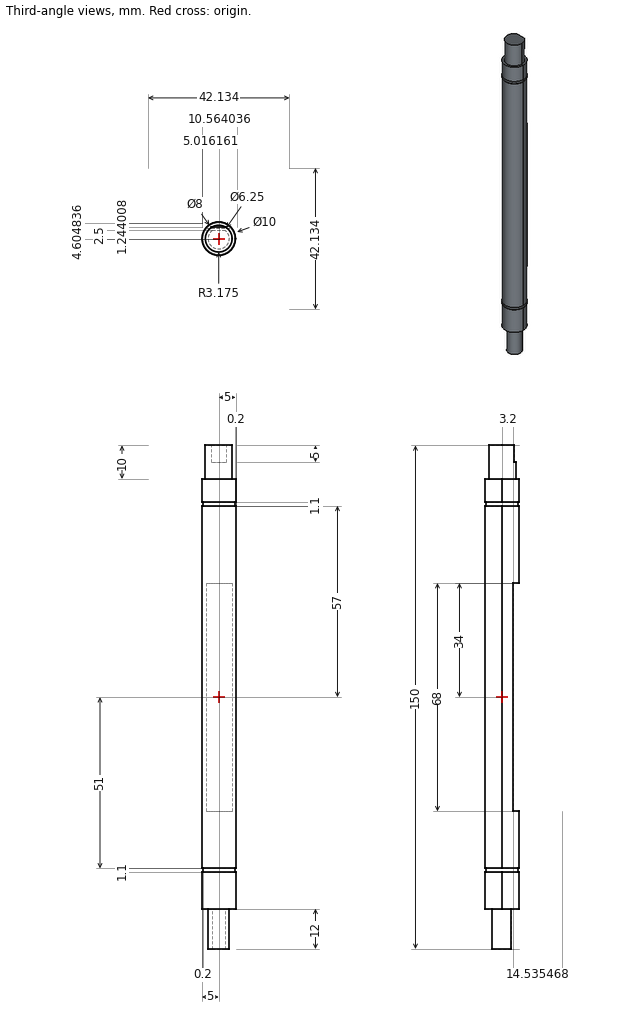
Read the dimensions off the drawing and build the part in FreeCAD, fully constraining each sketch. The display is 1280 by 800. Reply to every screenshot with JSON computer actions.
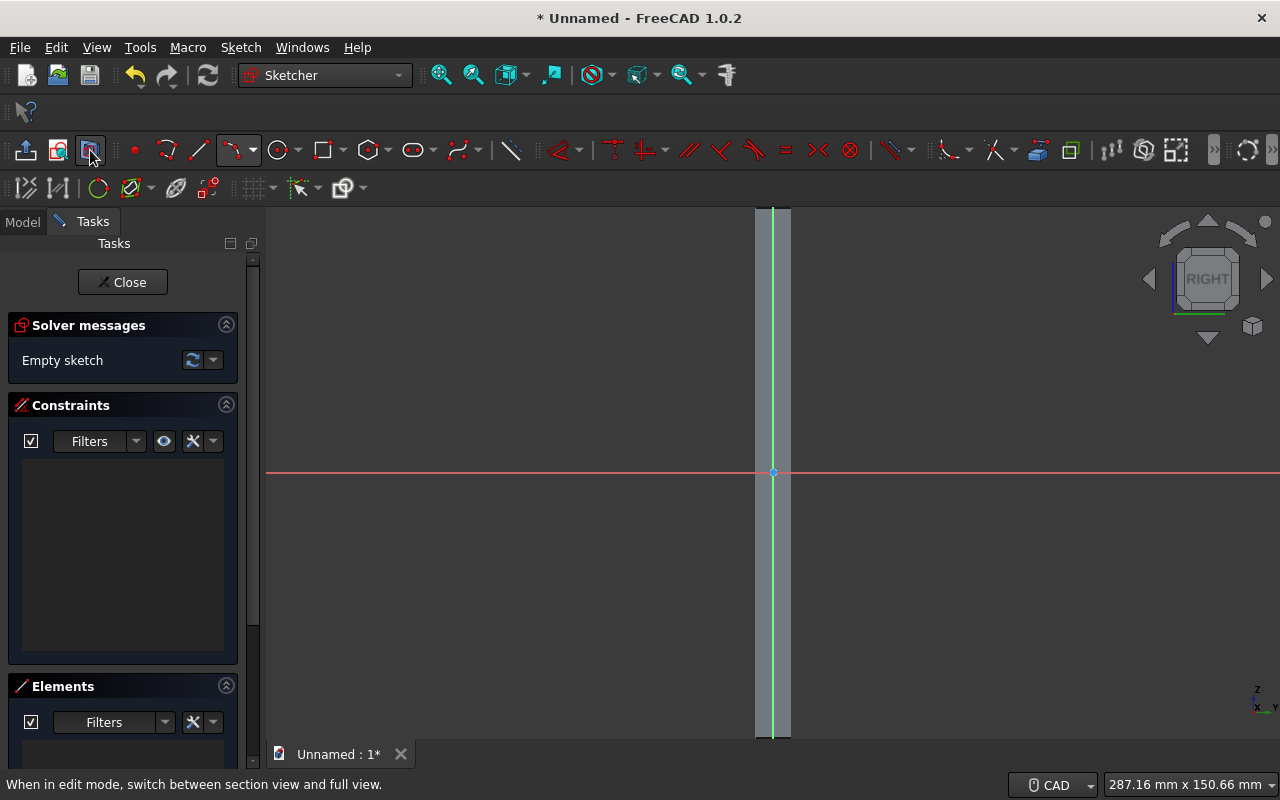
{"action": "scroll", "coordinate": [1007, 473], "scroll_direction": "up", "scroll_amount": 2}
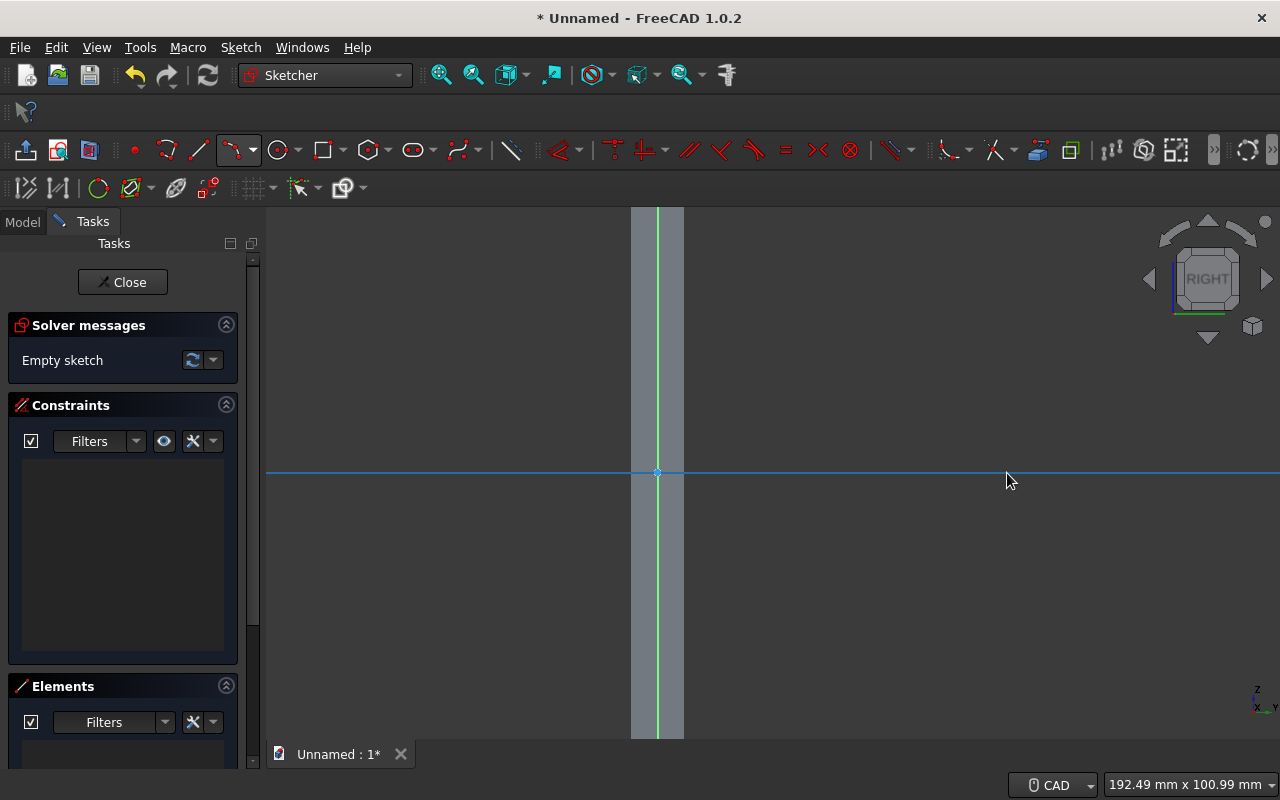
{"action": "key", "text": "g r"}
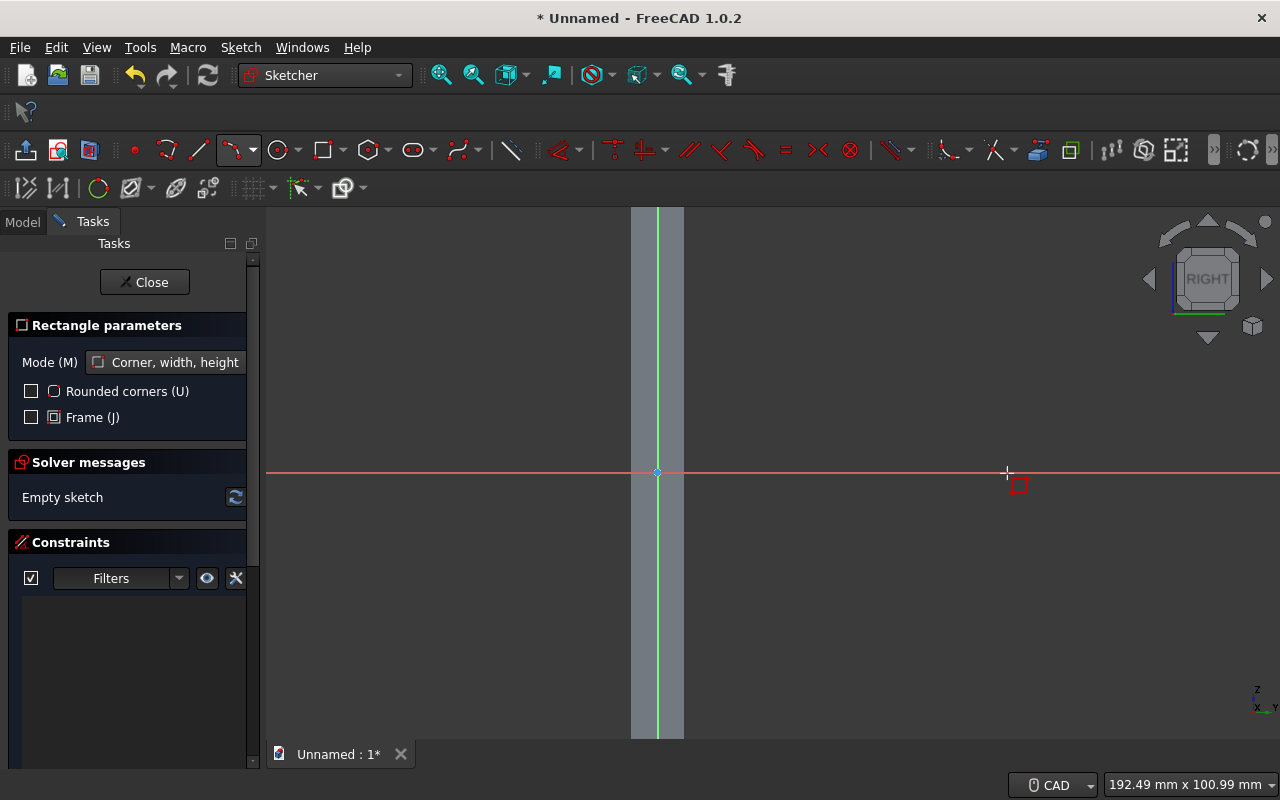
{"action": "left_click", "coordinate": [674, 294]}
{"action": "left_click", "coordinate": [751, 652]}
{"action": "key", "text": "Escape"}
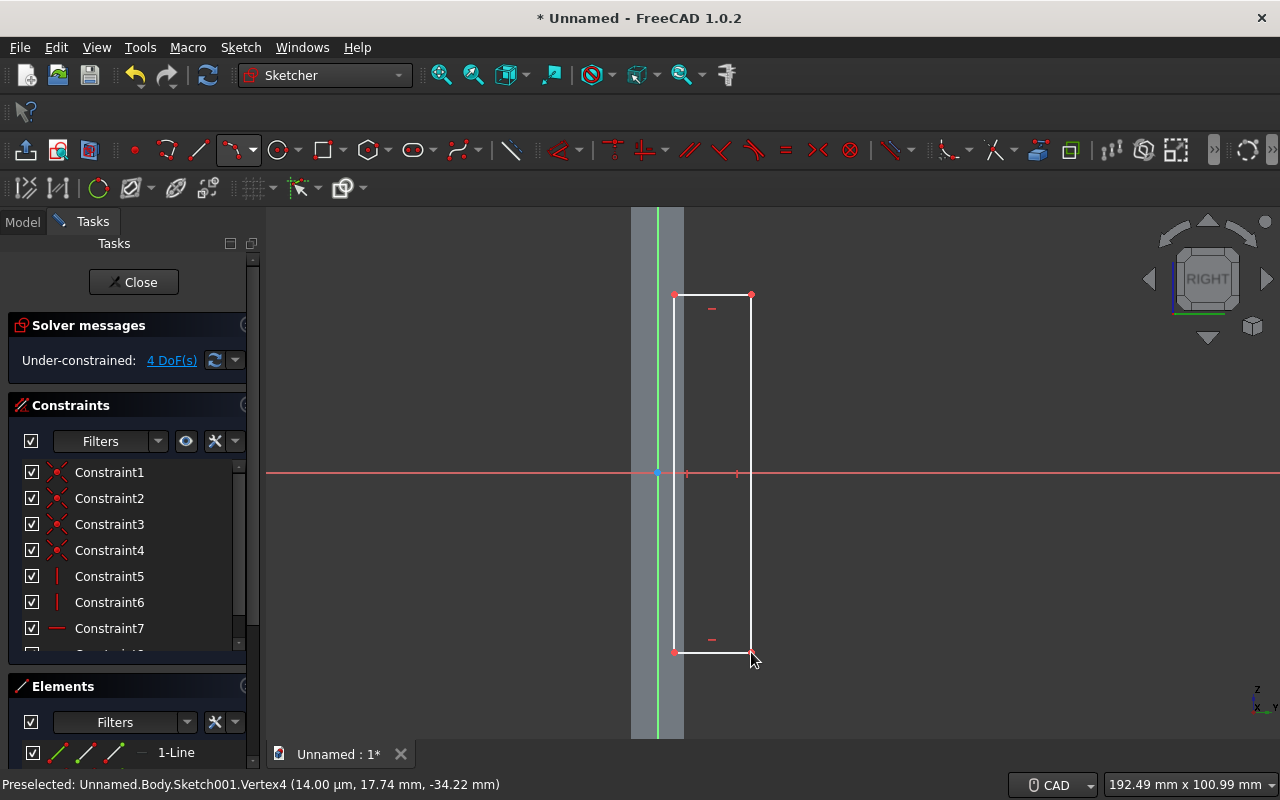
{"action": "left_click", "coordinate": [674, 402]}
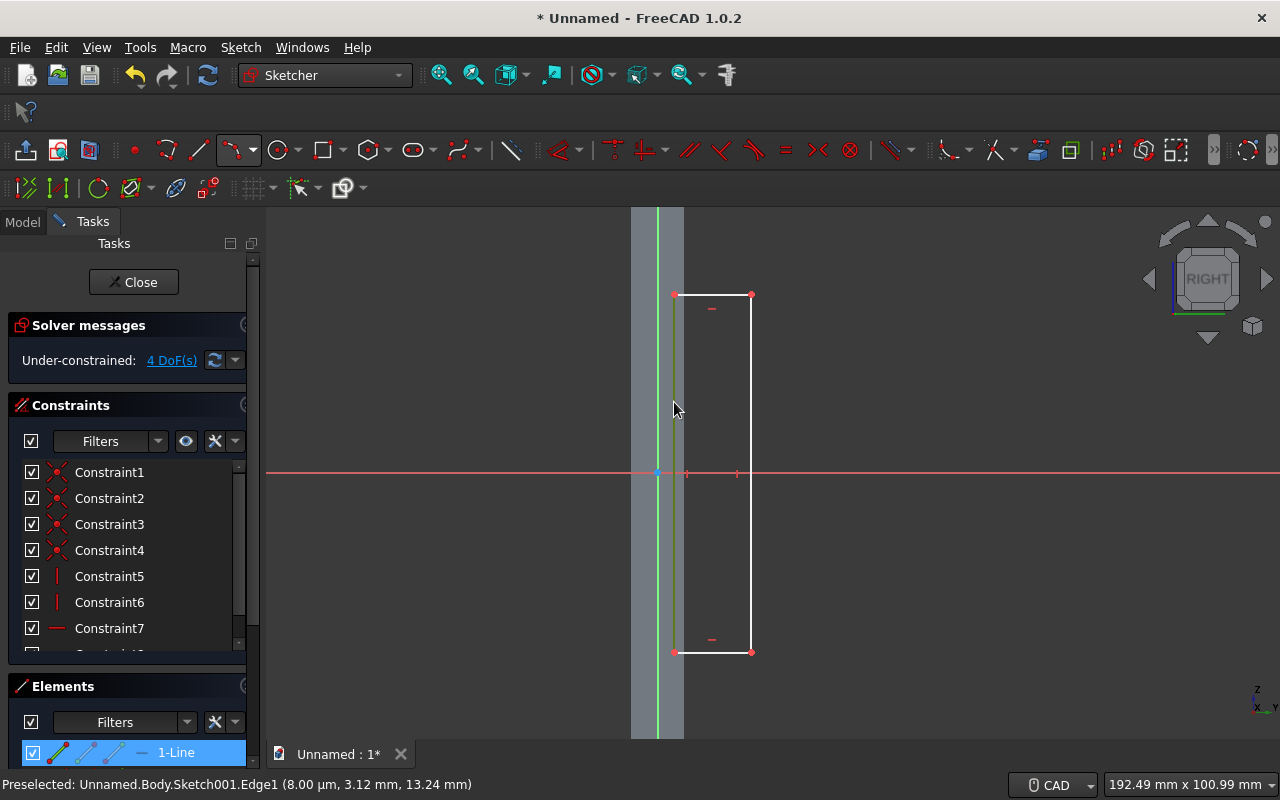
{"action": "key", "text": "i"}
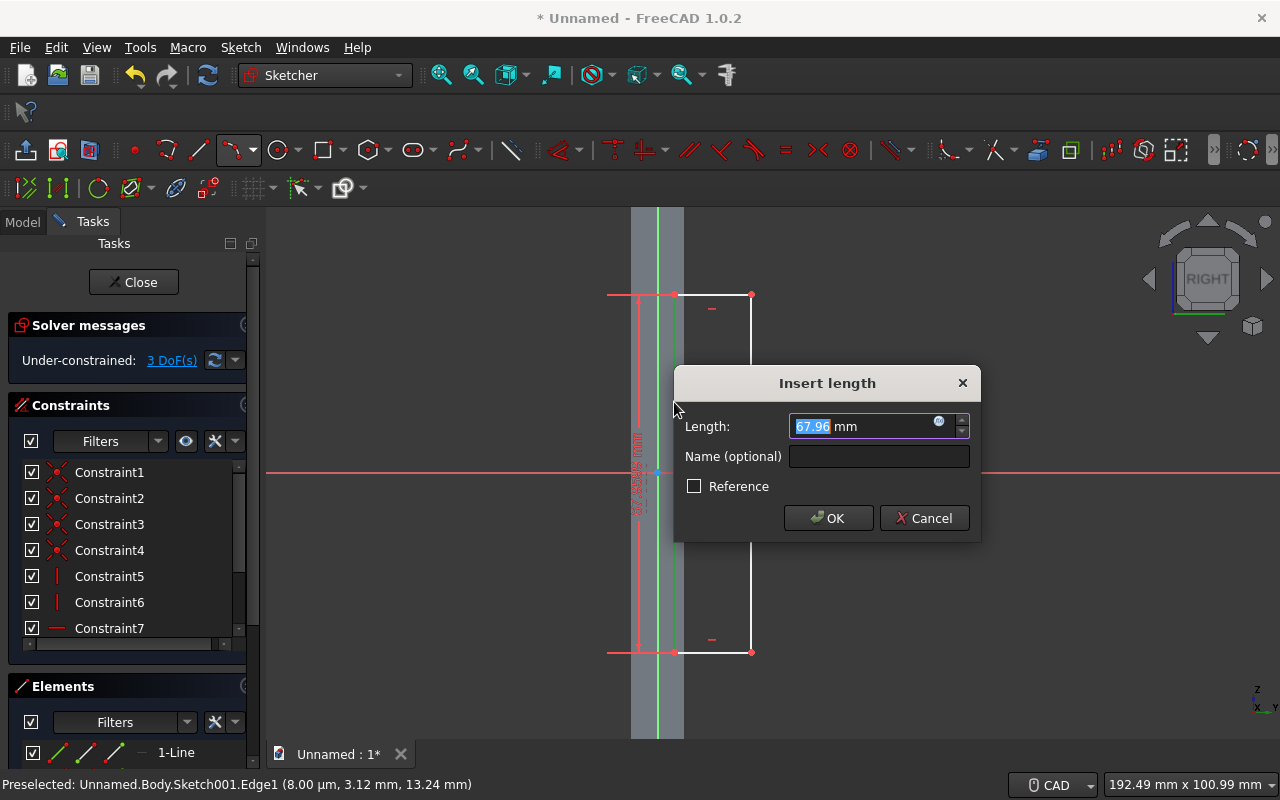
{"action": "type", "text": "68"}
{"action": "key", "text": "Return"}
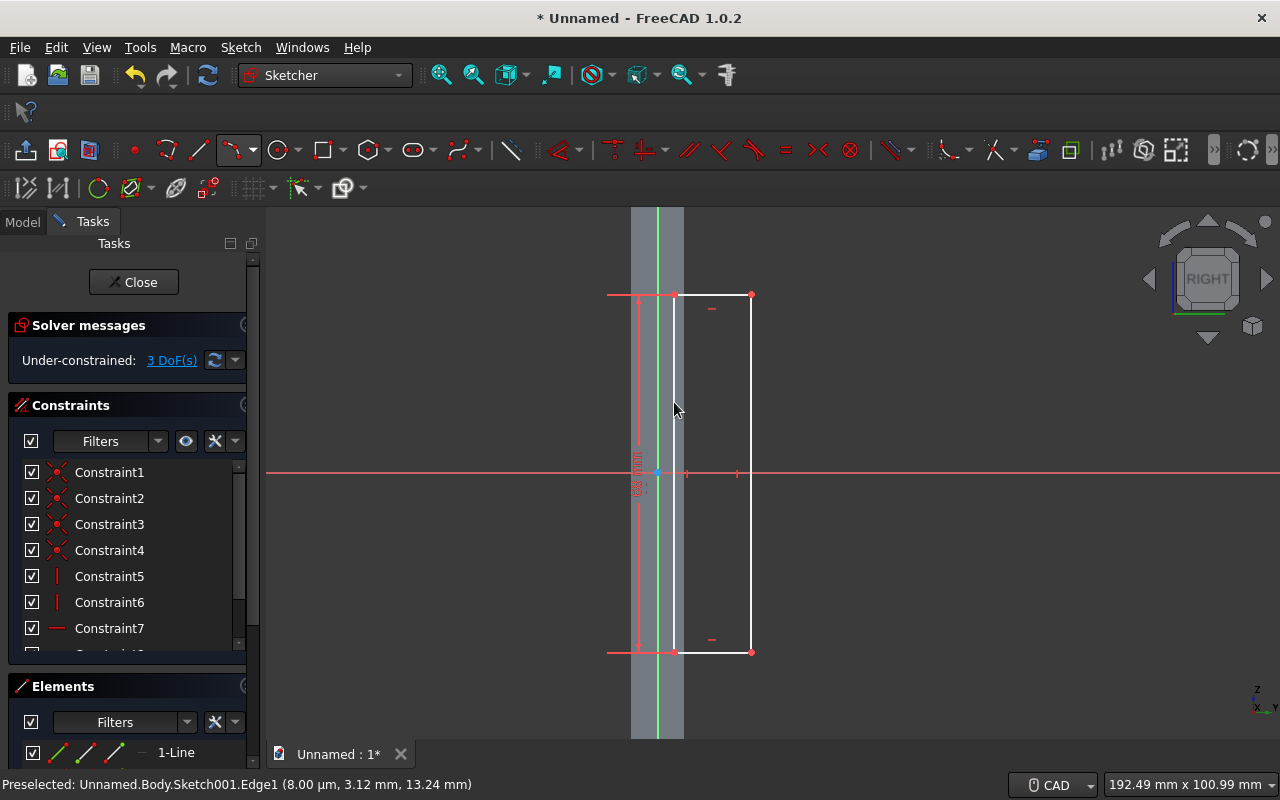
{"action": "left_click", "coordinate": [674, 295]}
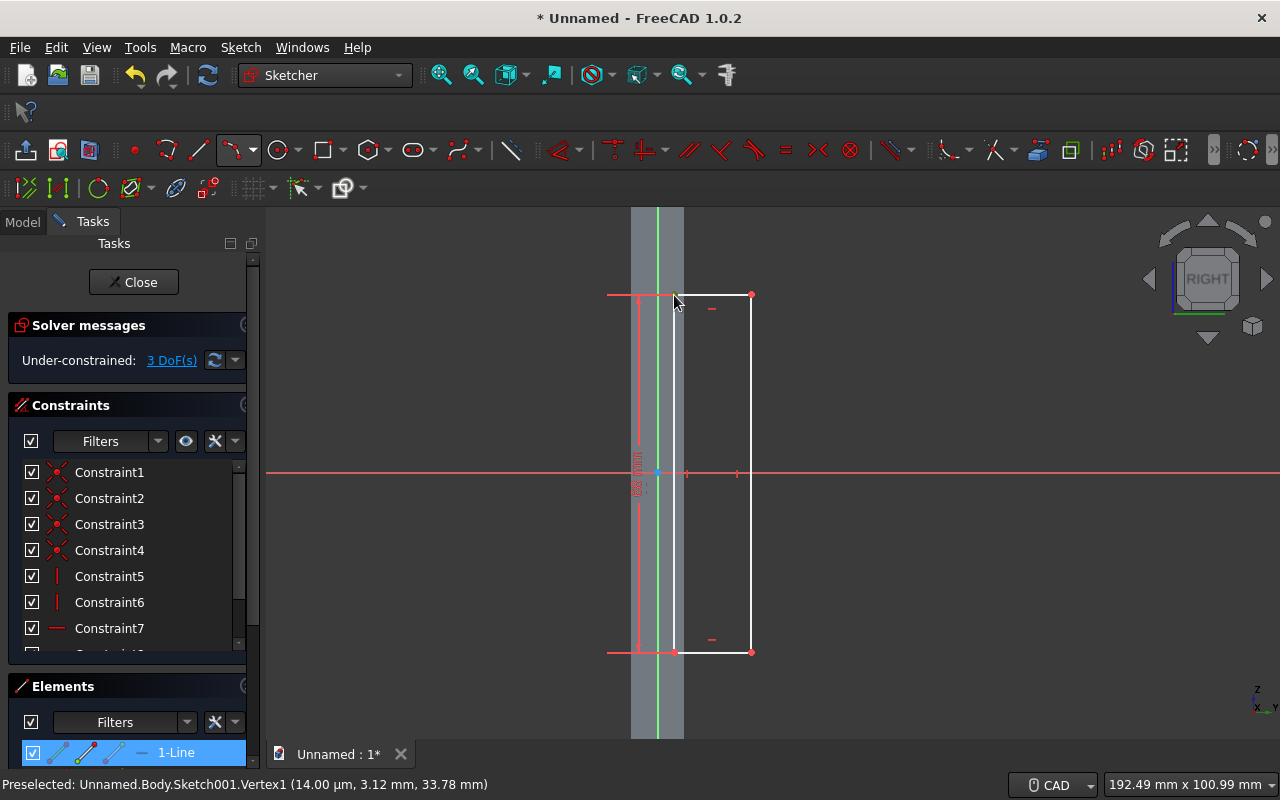
{"action": "left_click", "coordinate": [582, 150]}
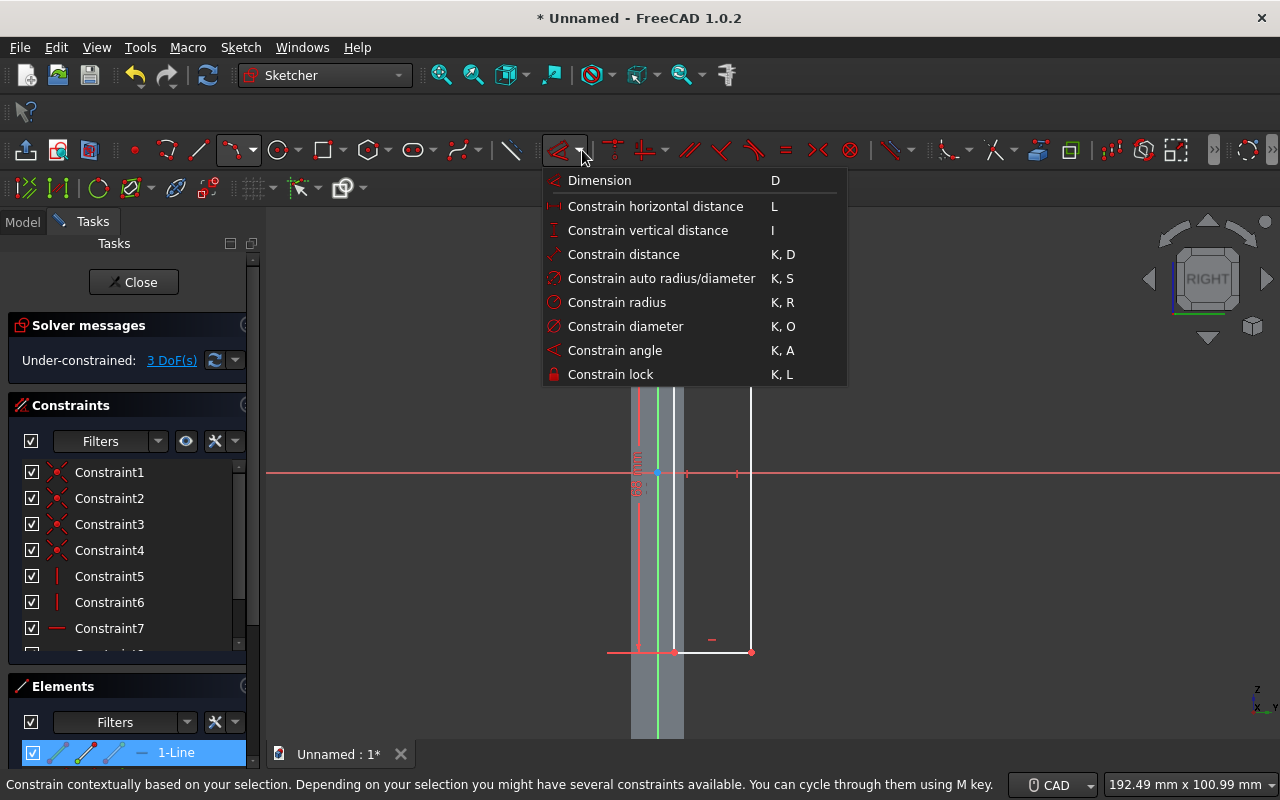
{"action": "left_click", "coordinate": [695, 230]}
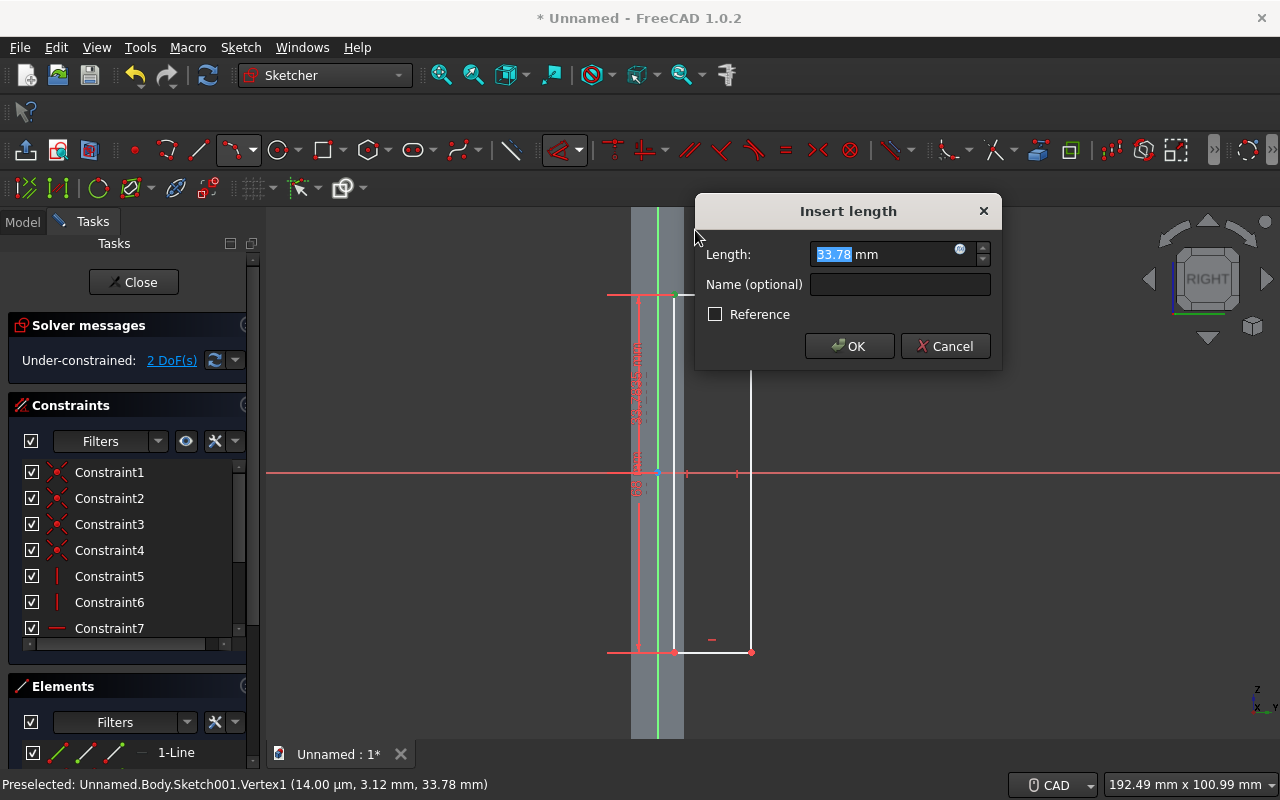
{"action": "type", "text": "34"}
{"action": "key", "text": "Return"}